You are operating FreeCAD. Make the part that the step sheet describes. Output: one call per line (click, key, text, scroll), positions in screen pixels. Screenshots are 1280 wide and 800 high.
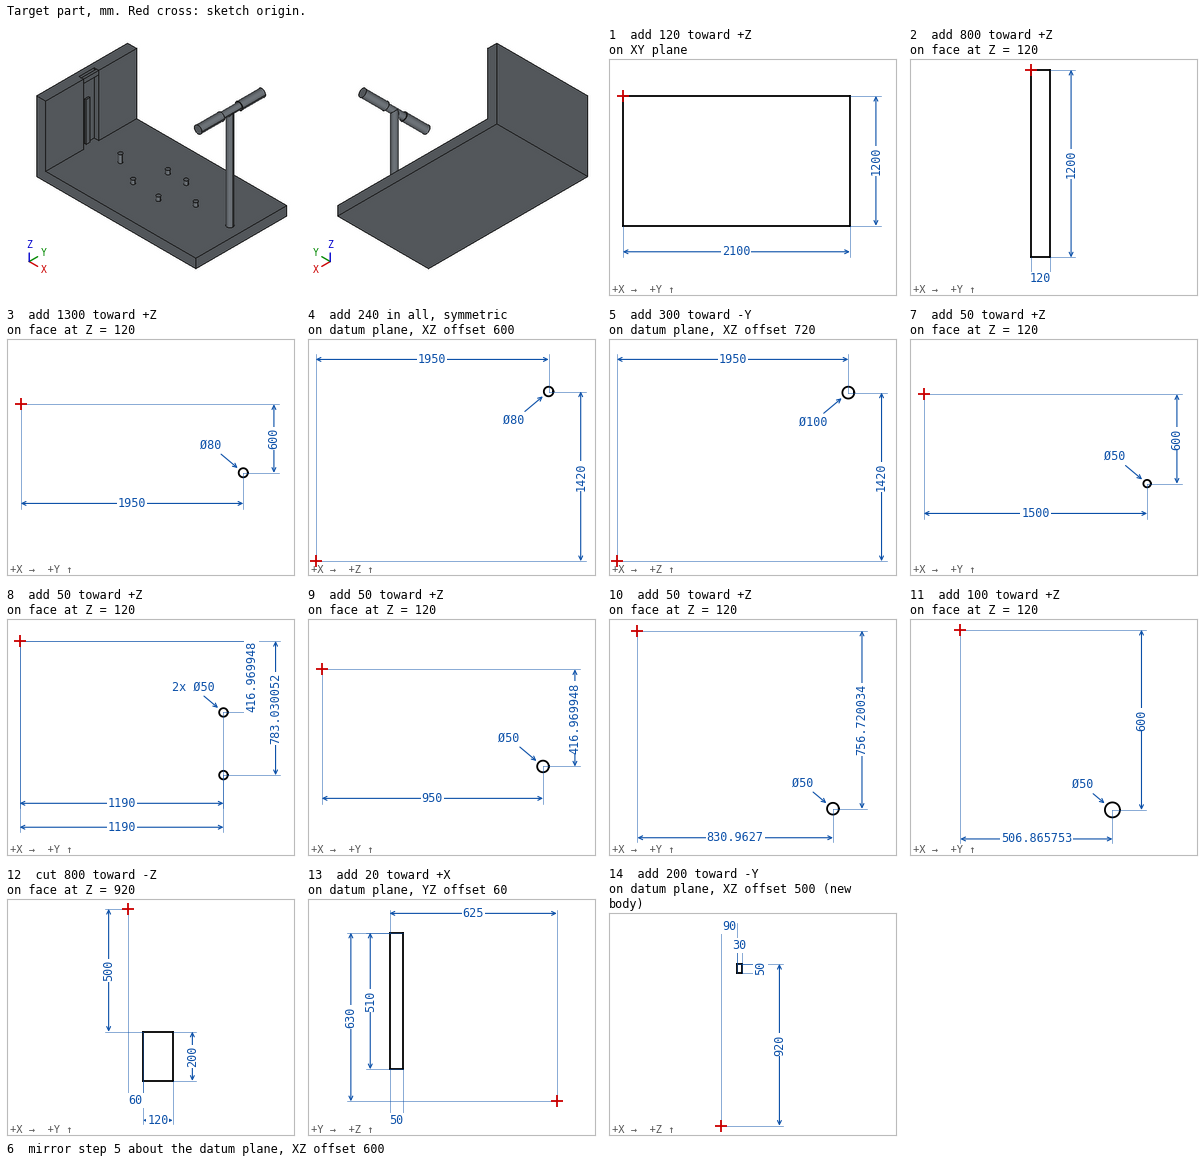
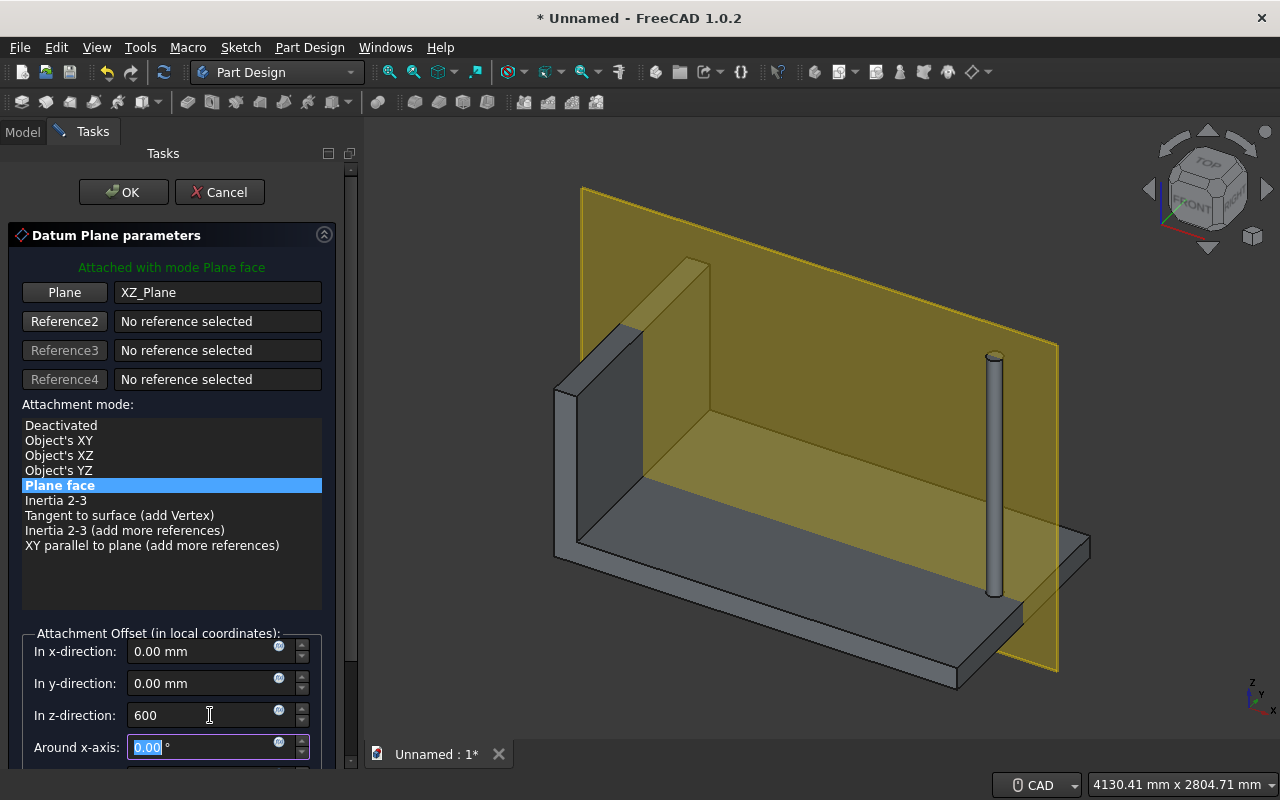
click(124, 192)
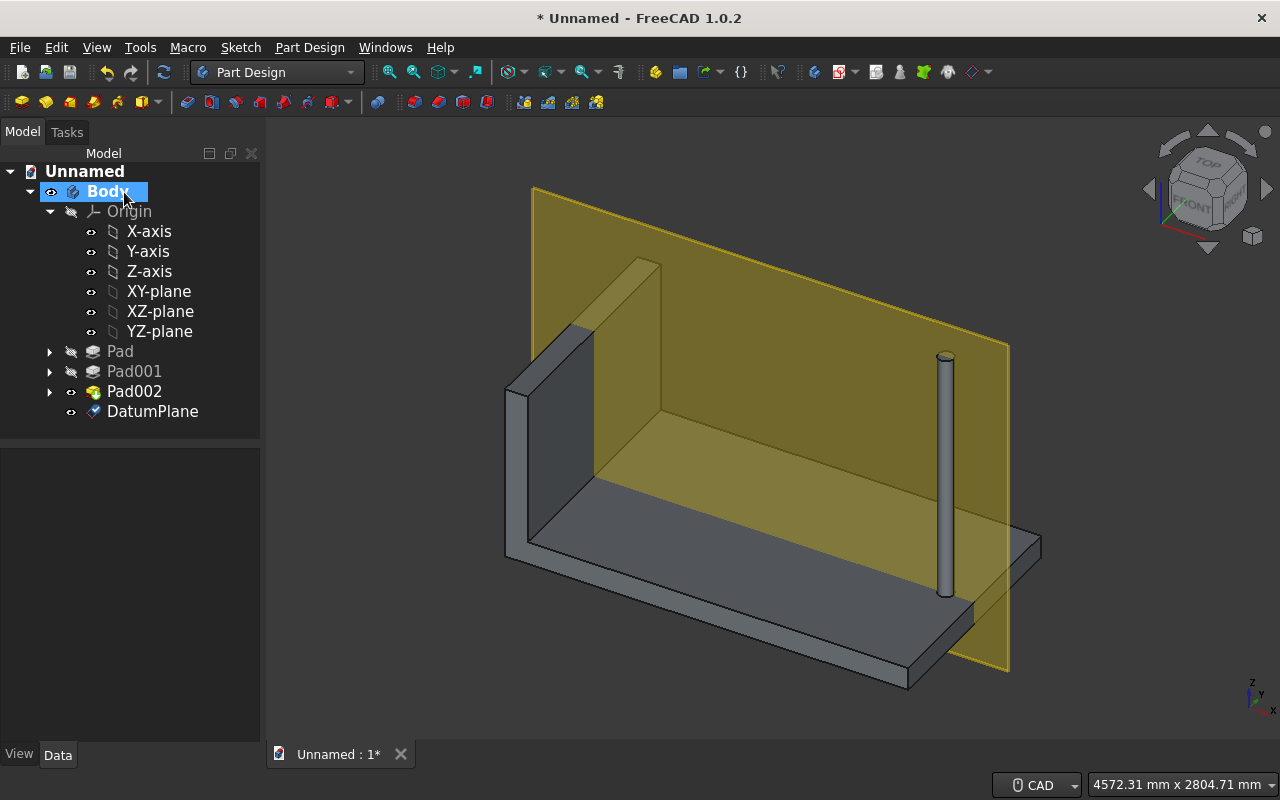
click(116, 412)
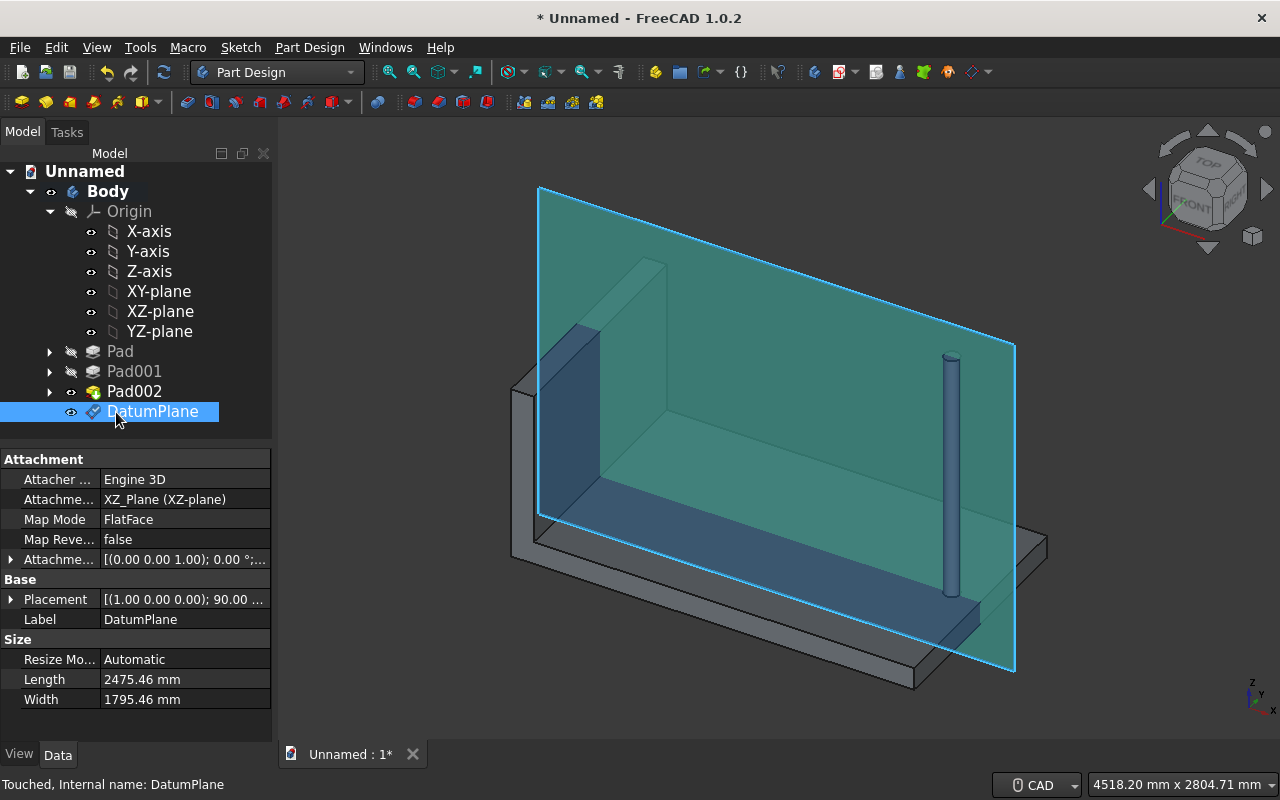
click(840, 72)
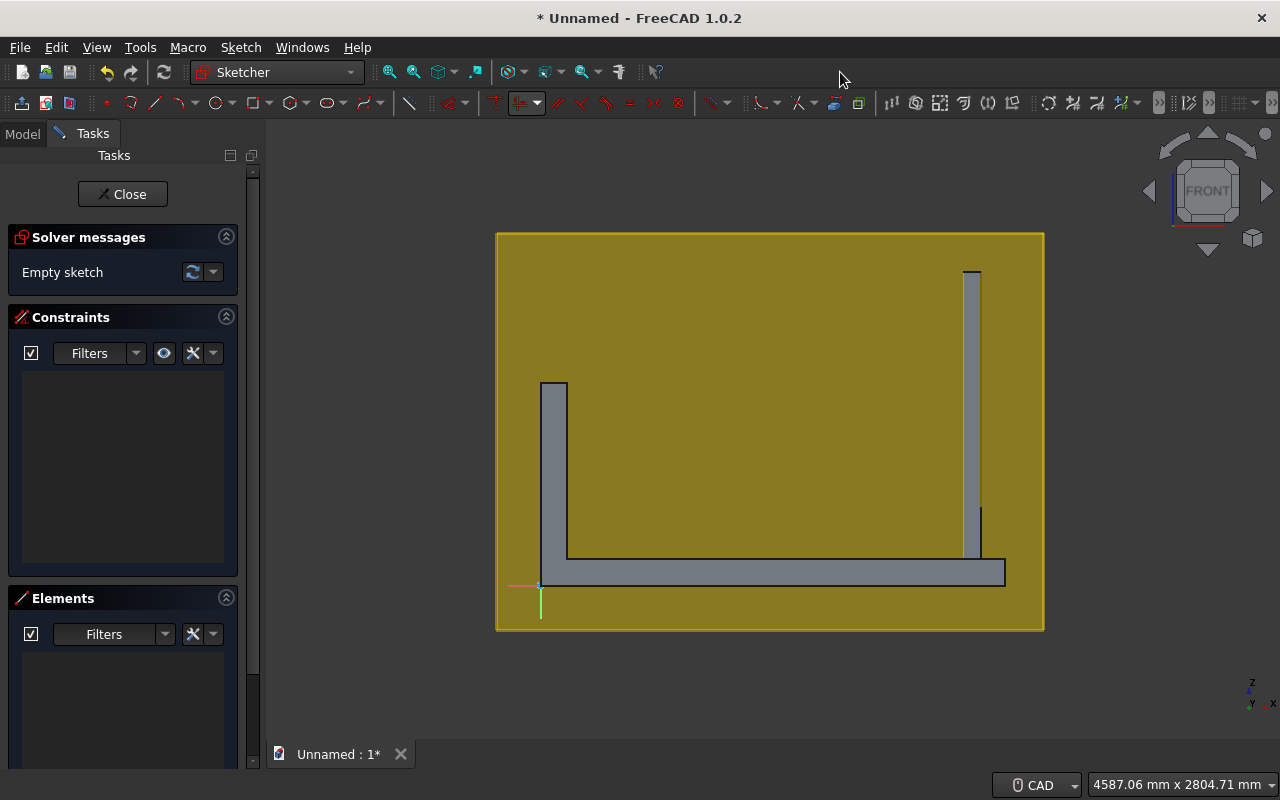
click(70, 104)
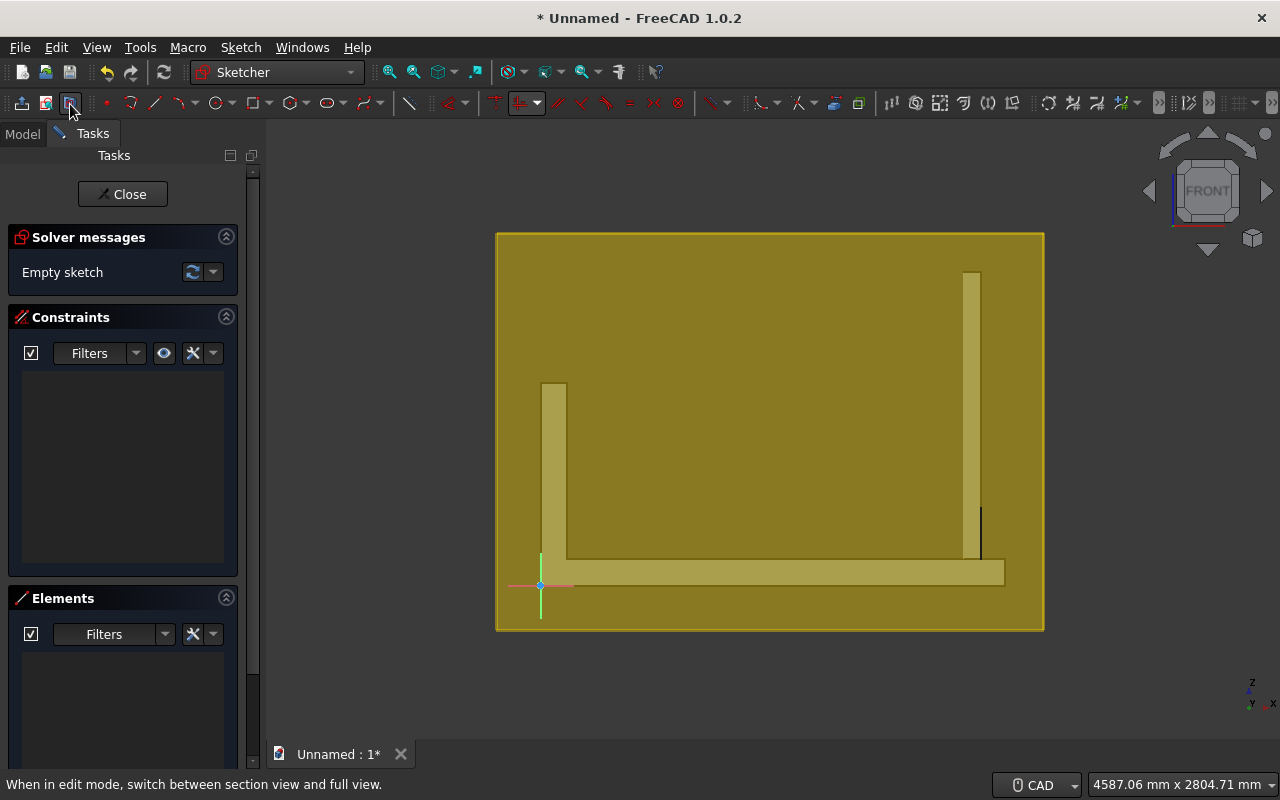
scroll(986, 264, up, 15)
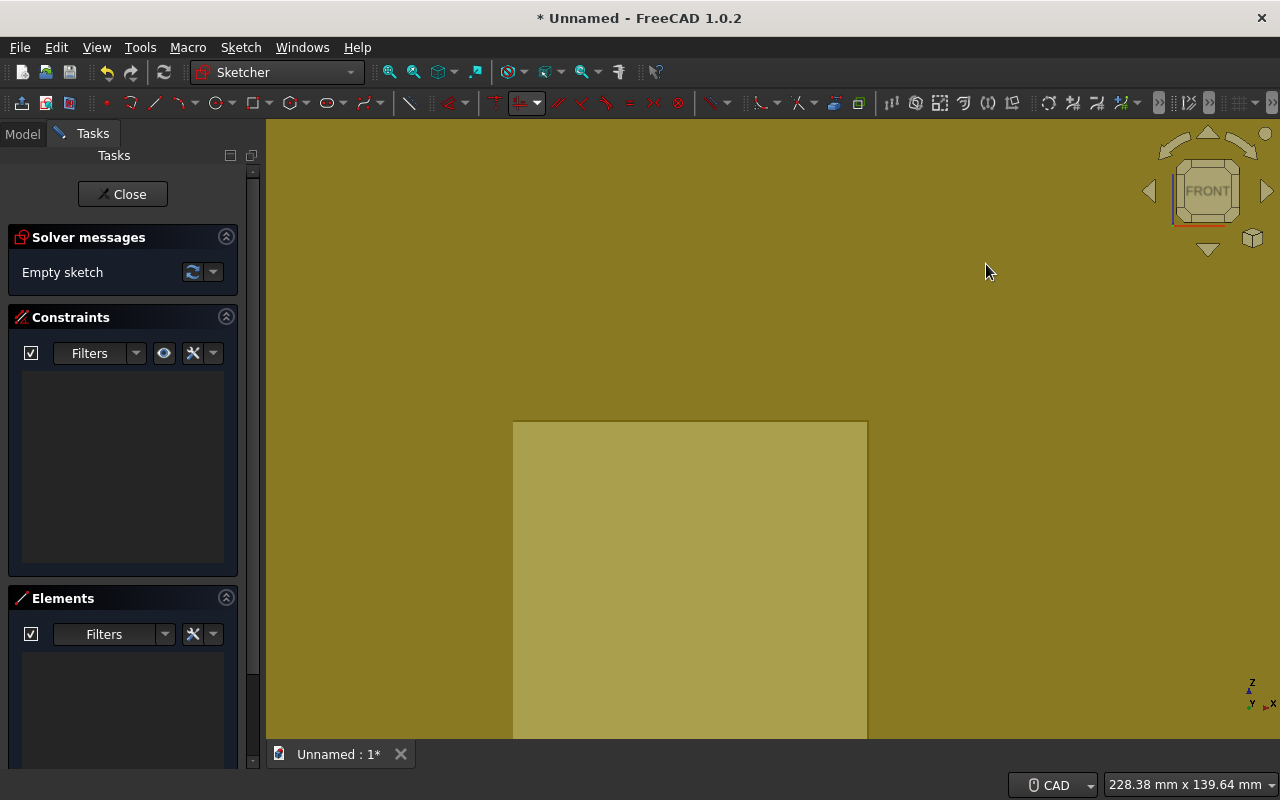
key(g)
key(c)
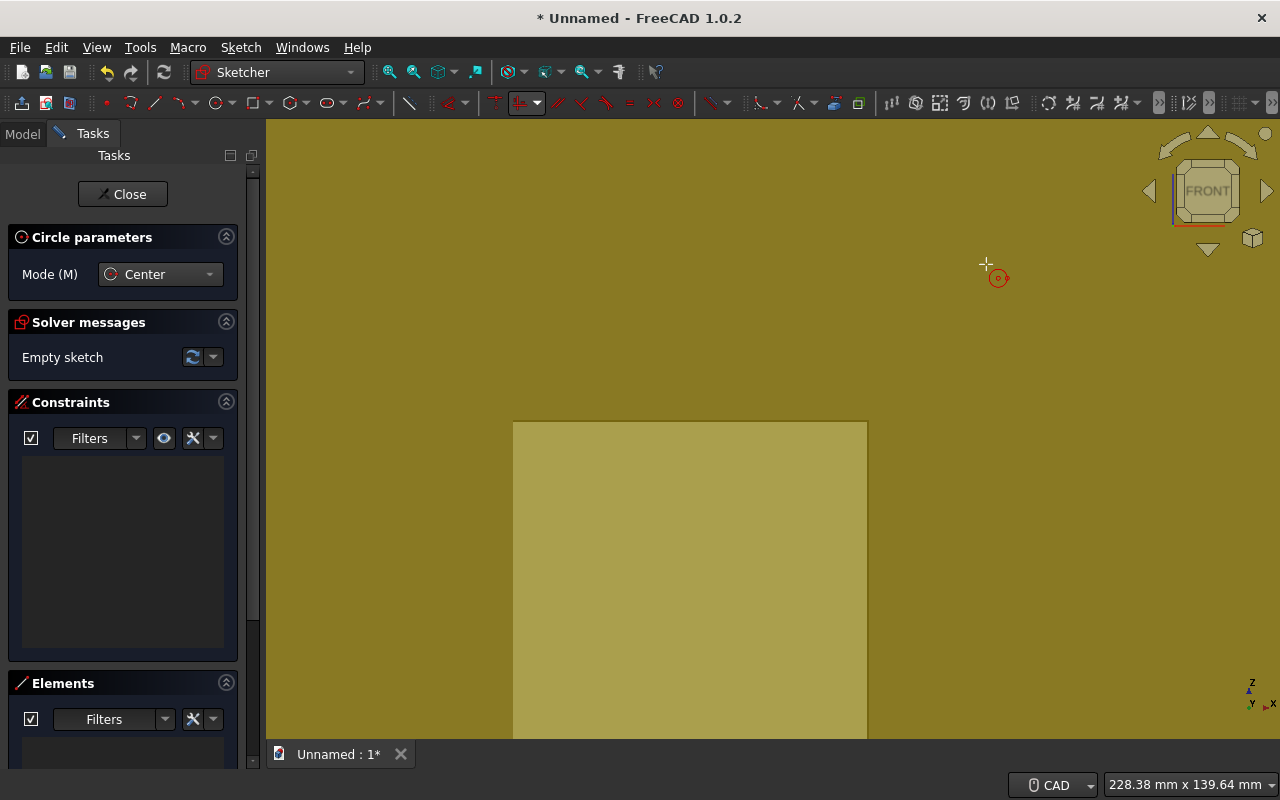
click(690, 421)
move(816, 296)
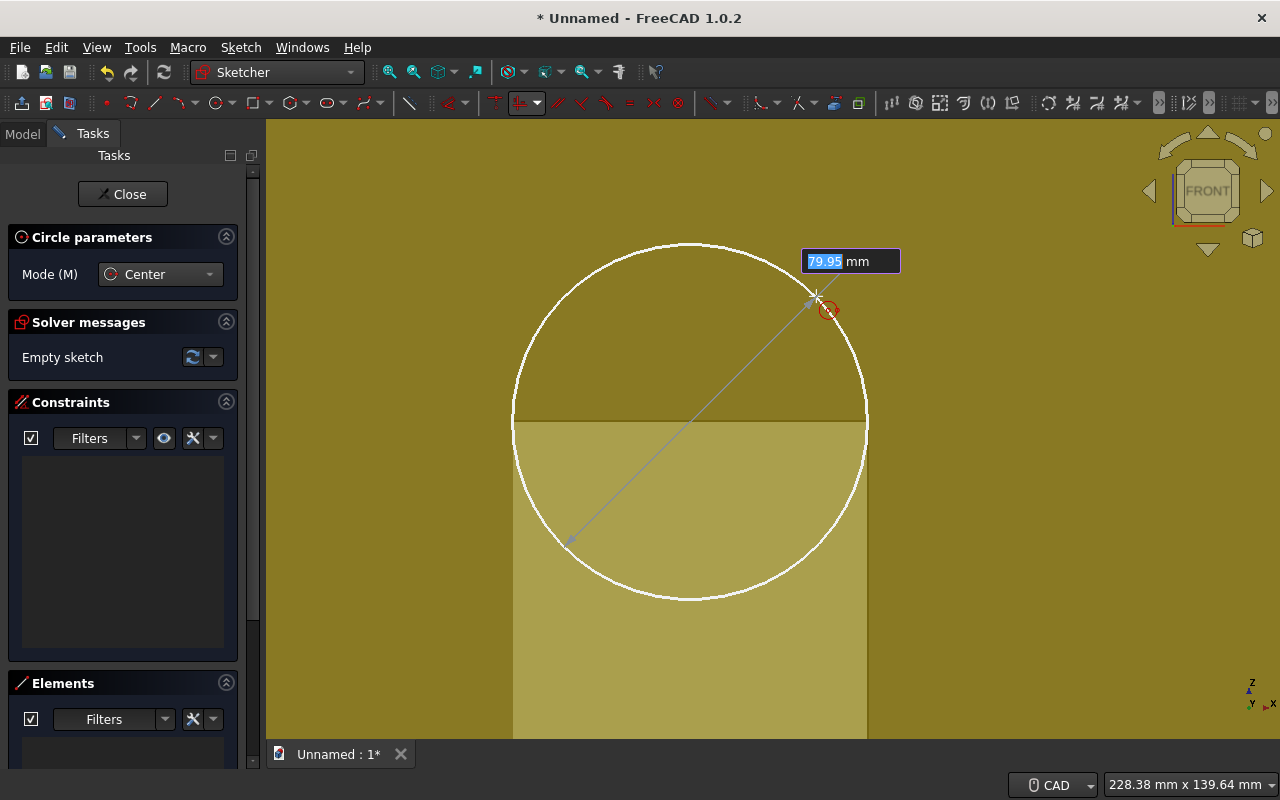
text(80)
key(Return)
key(Escape)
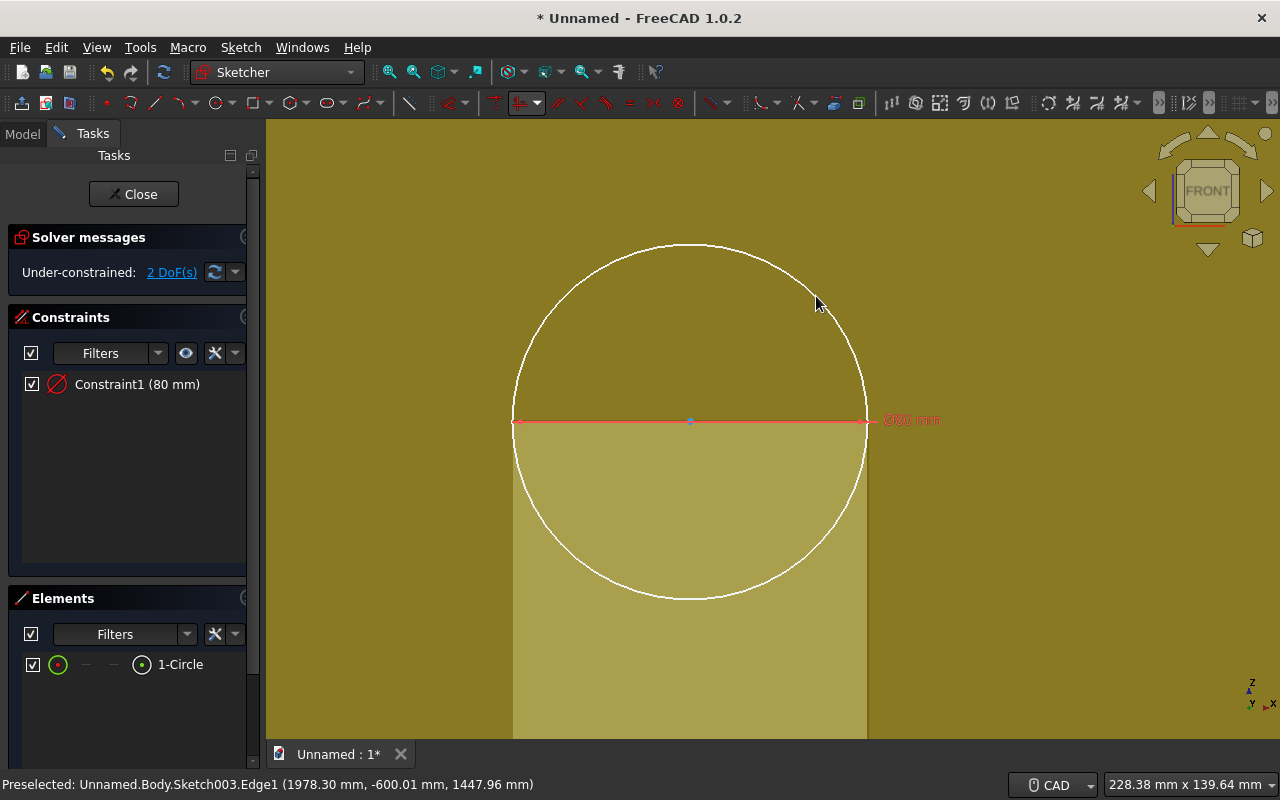
click(448, 104)